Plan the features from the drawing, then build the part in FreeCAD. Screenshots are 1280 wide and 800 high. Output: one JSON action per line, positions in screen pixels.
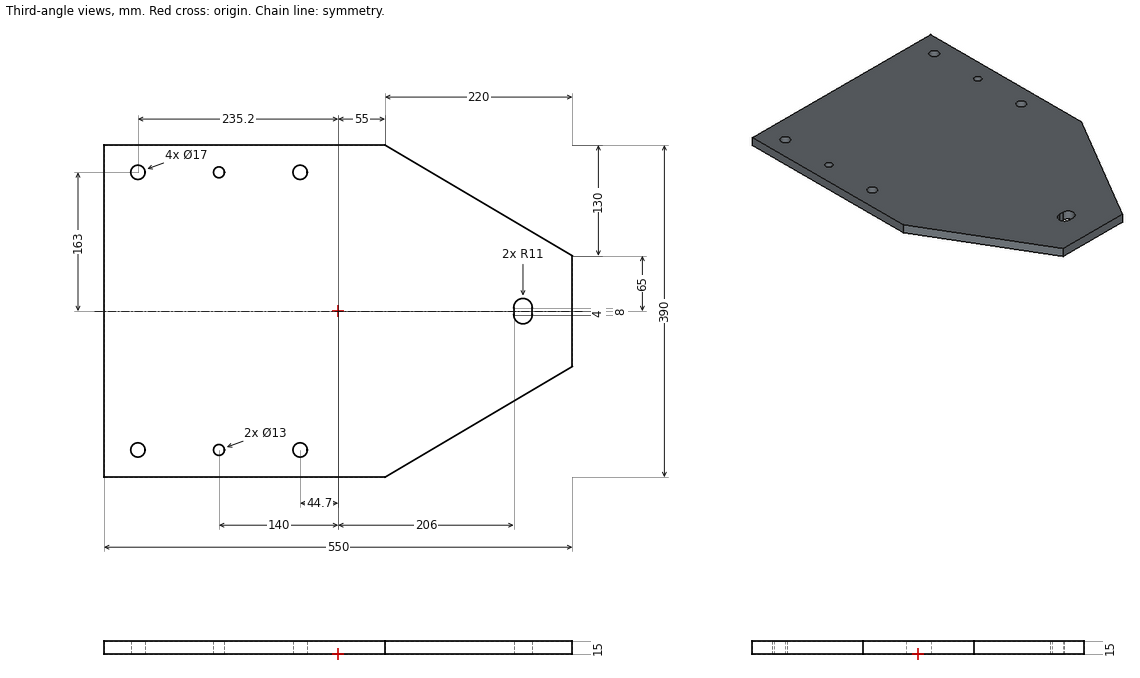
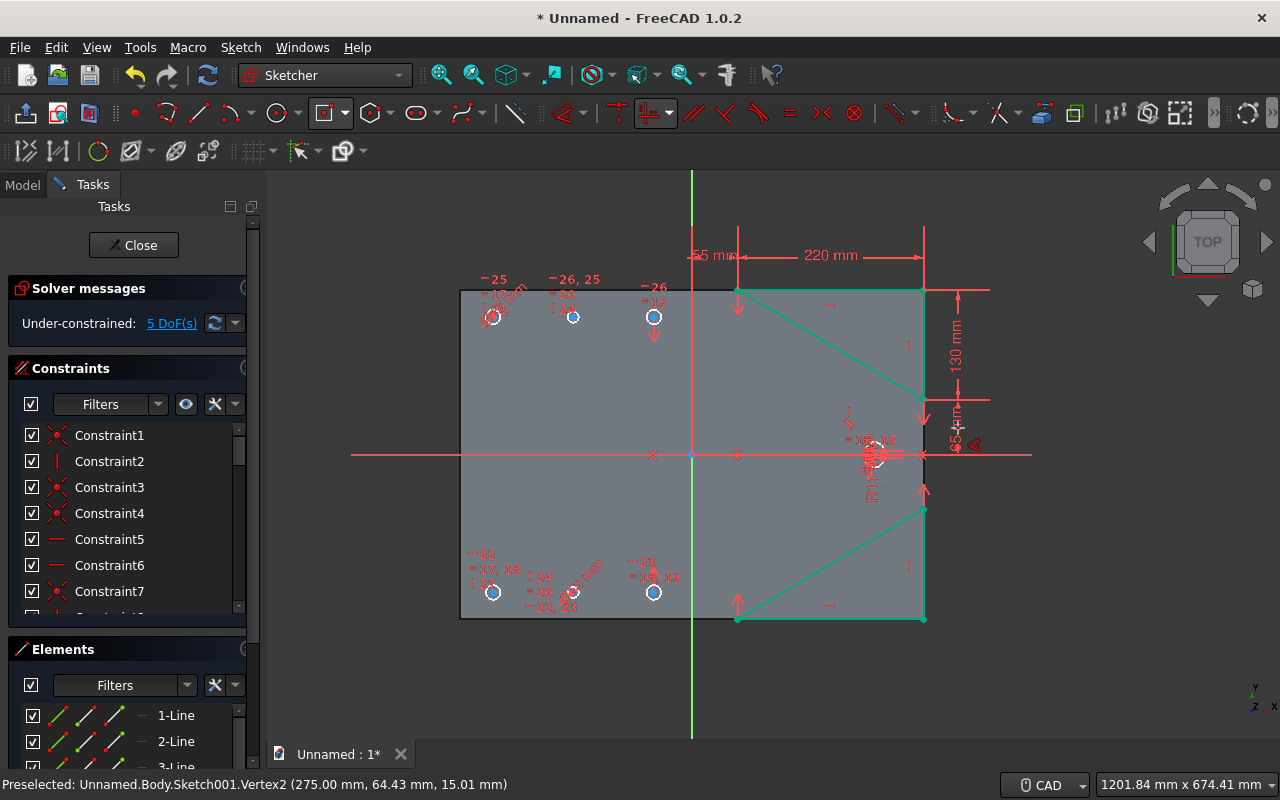
{"action": "left_click", "coordinate": [493, 317]}
{"action": "left_click", "coordinate": [459, 386]}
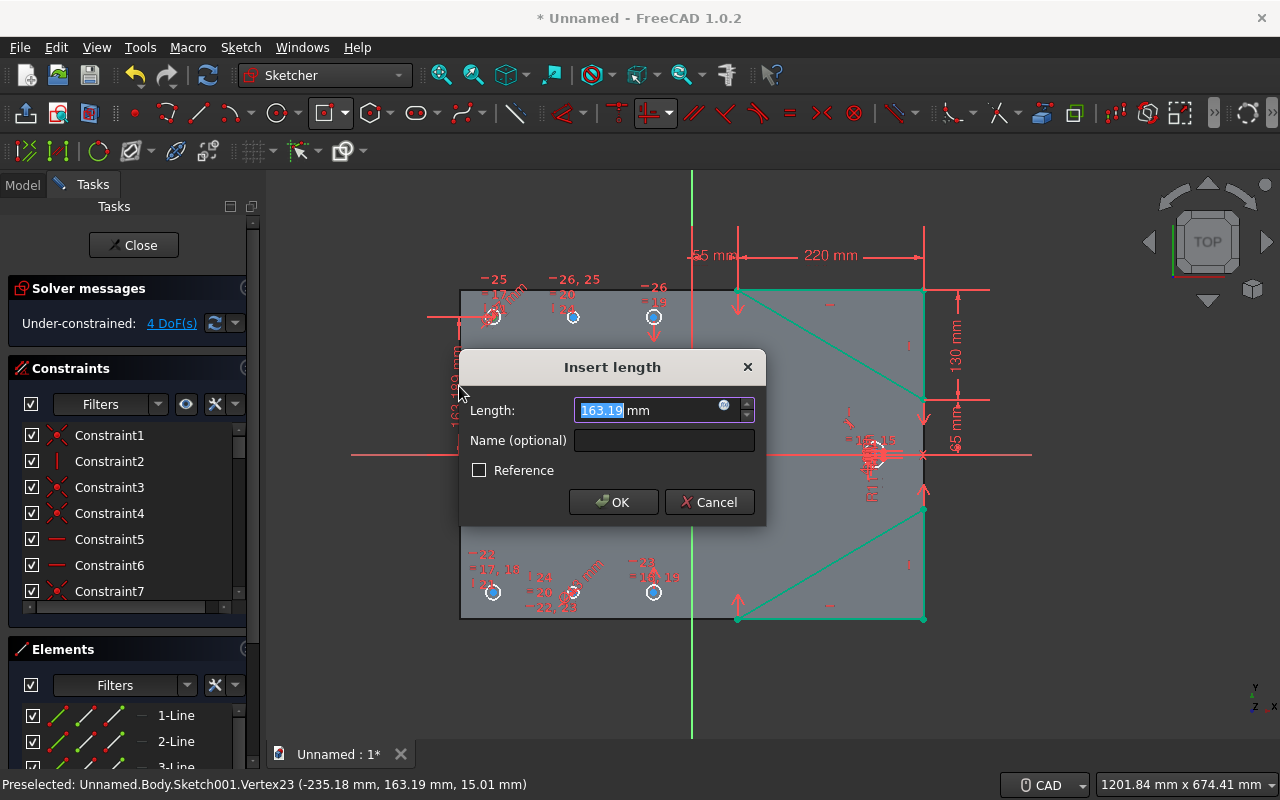
{"action": "type", "text": "163"}
{"action": "key", "text": "Return"}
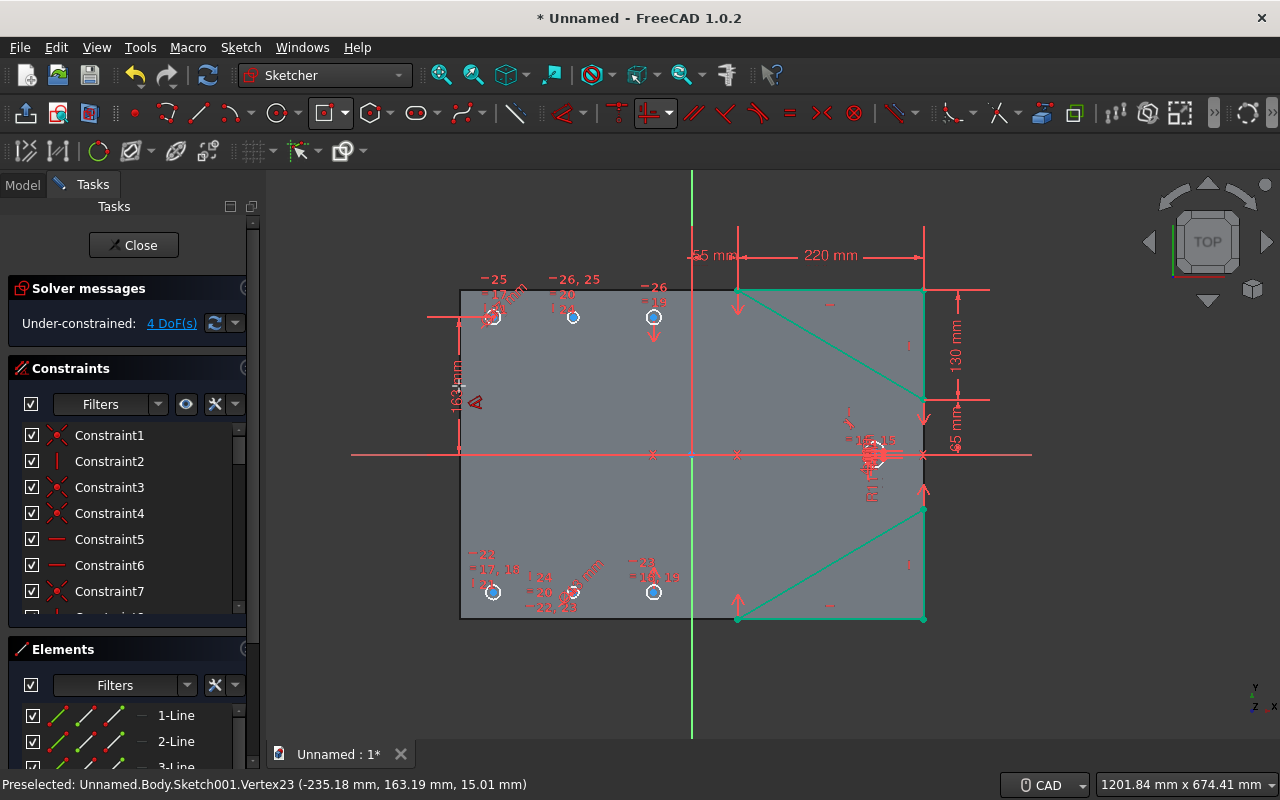
{"action": "left_click", "coordinate": [573, 592]}
{"action": "left_click", "coordinate": [632, 626]}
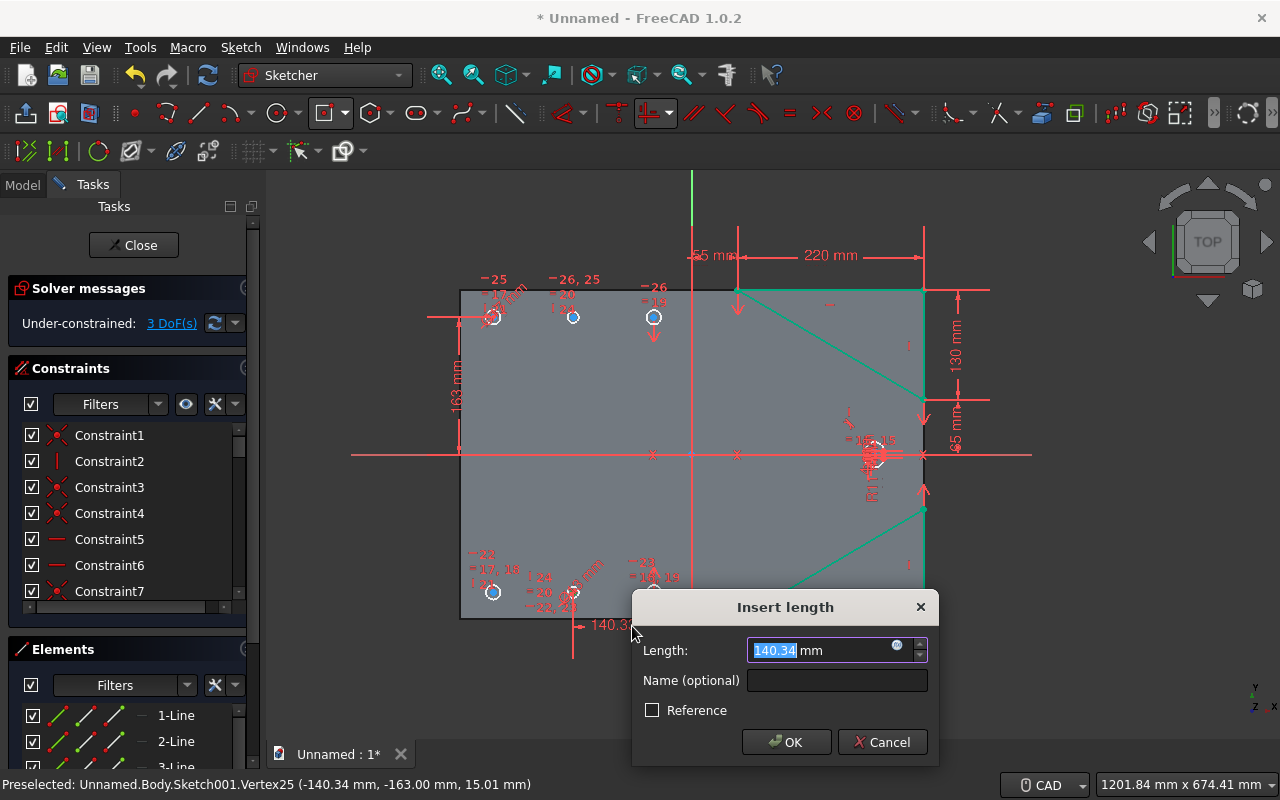
{"action": "type", "text": "140"}
{"action": "key", "text": "Return"}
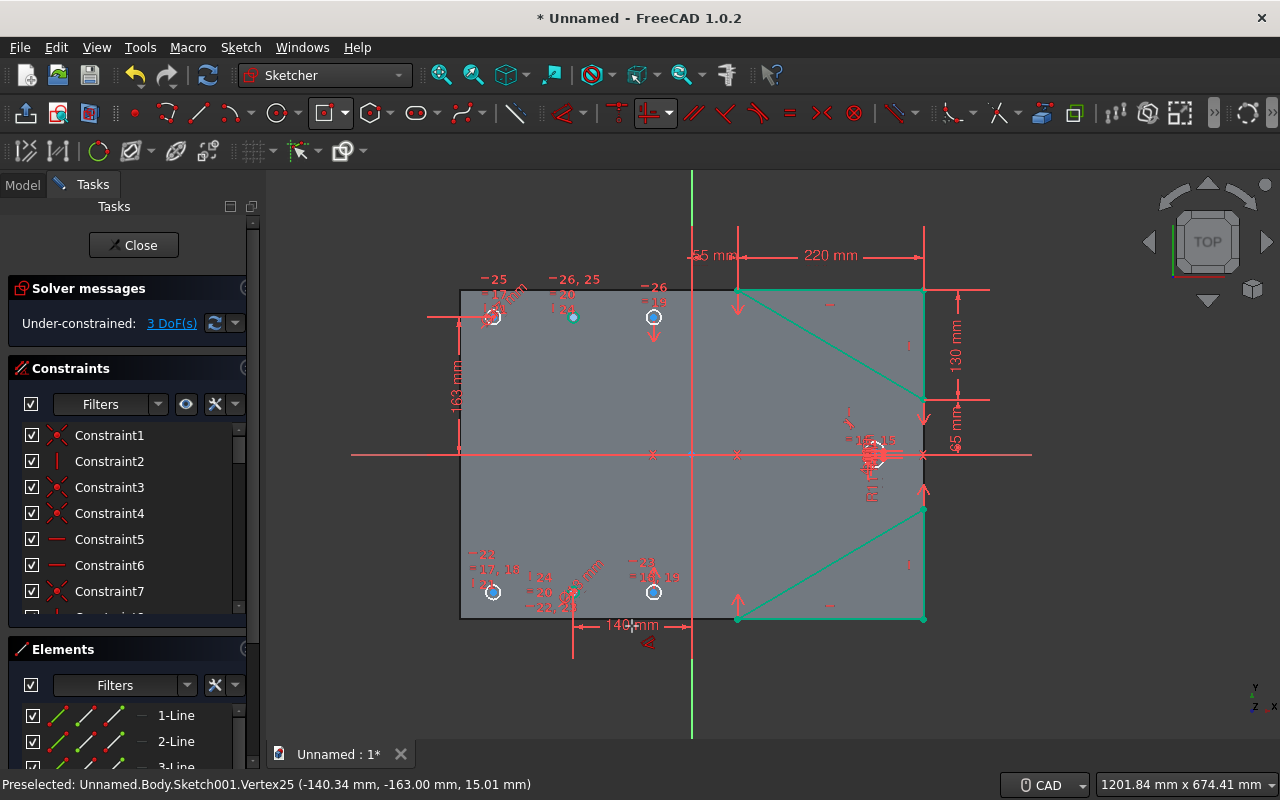
{"action": "scroll", "coordinate": [865, 458], "scroll_direction": "up", "scroll_amount": 3}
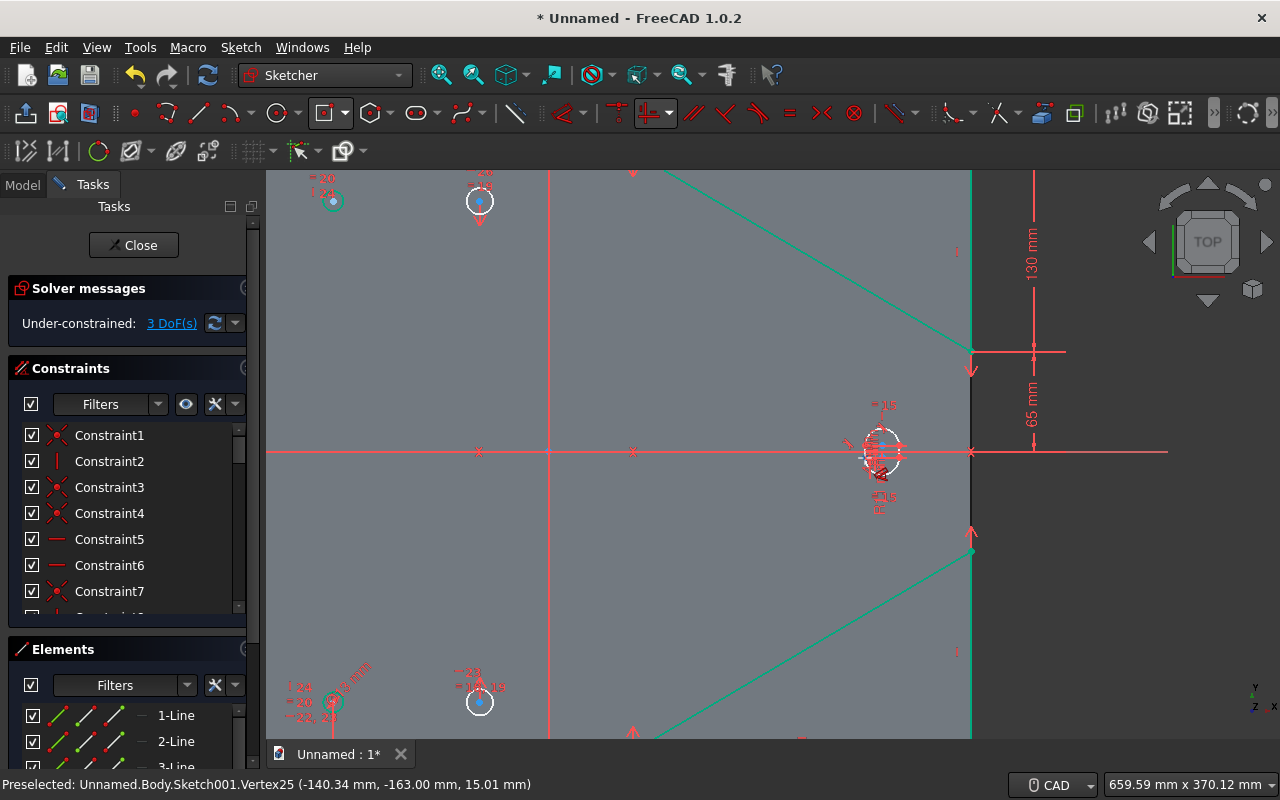
{"action": "left_click", "coordinate": [865, 458]}
{"action": "left_click", "coordinate": [707, 492]}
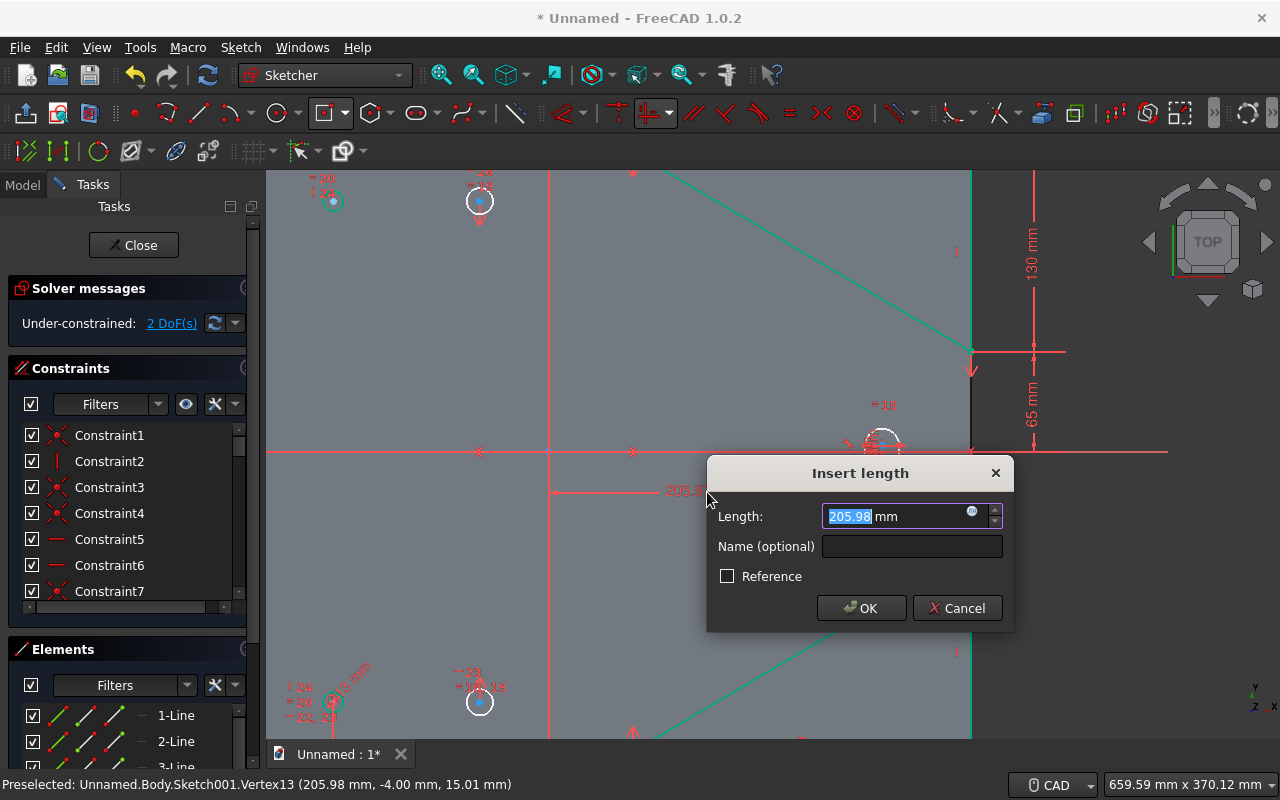
{"action": "type", "text": "206"}
{"action": "key", "text": "Return"}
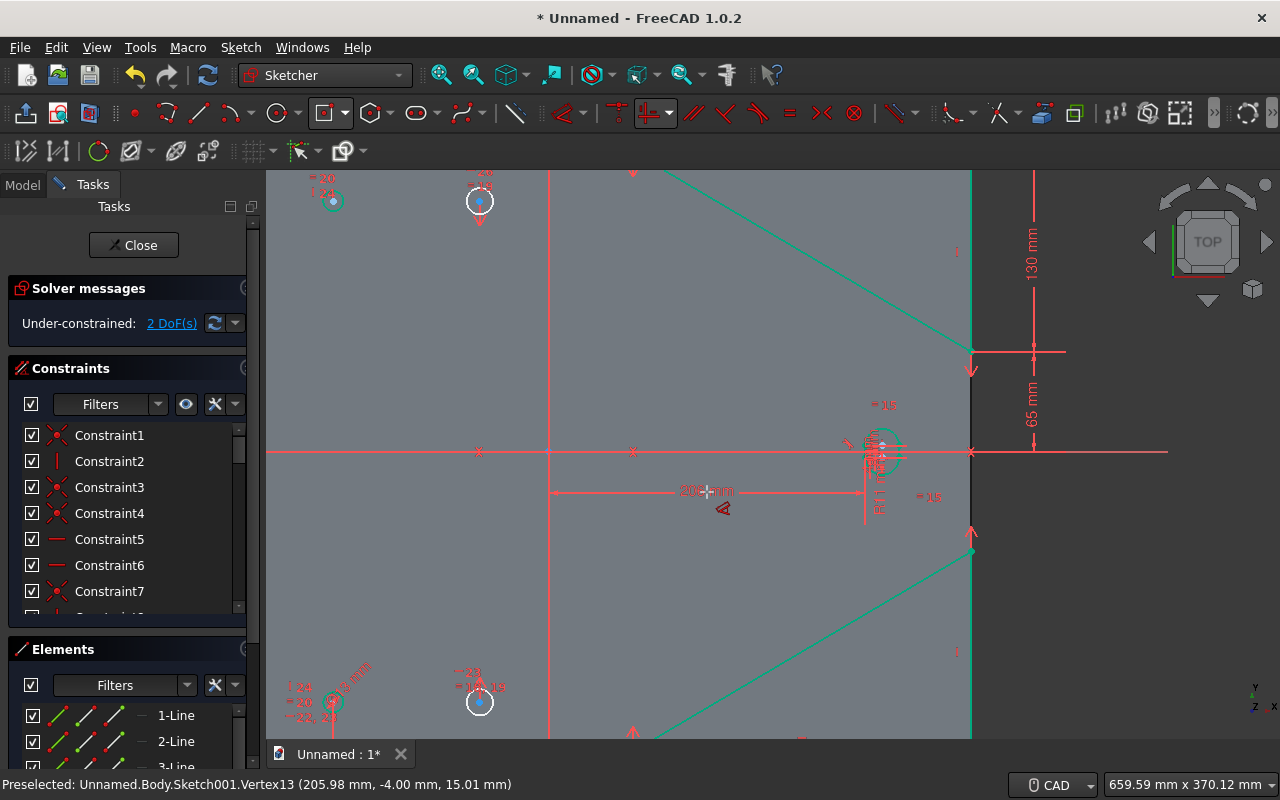
{"action": "left_click", "coordinate": [480, 702]}
{"action": "left_click", "coordinate": [514, 418]}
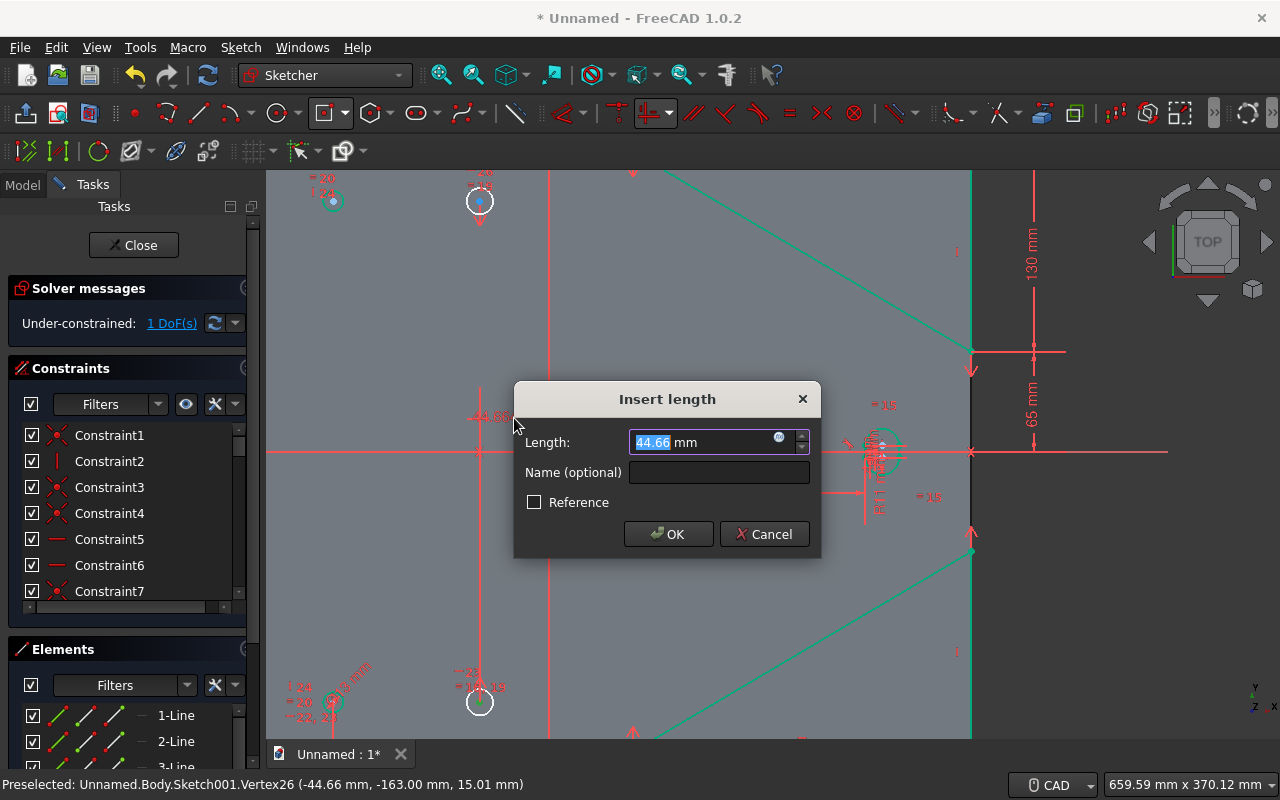
{"action": "type", "text": "44.7"}
{"action": "key", "text": "Return"}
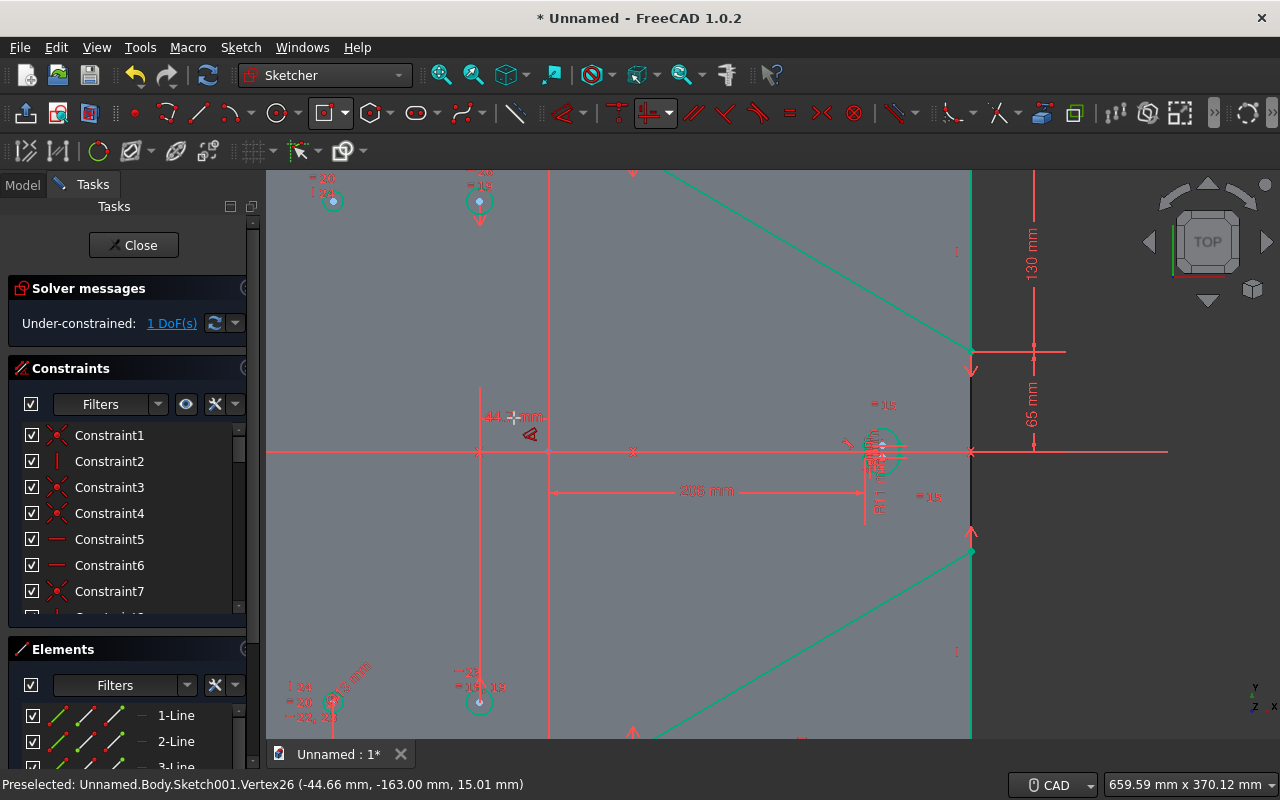
{"action": "scroll", "coordinate": [865, 458], "scroll_direction": "down", "scroll_amount": 3}